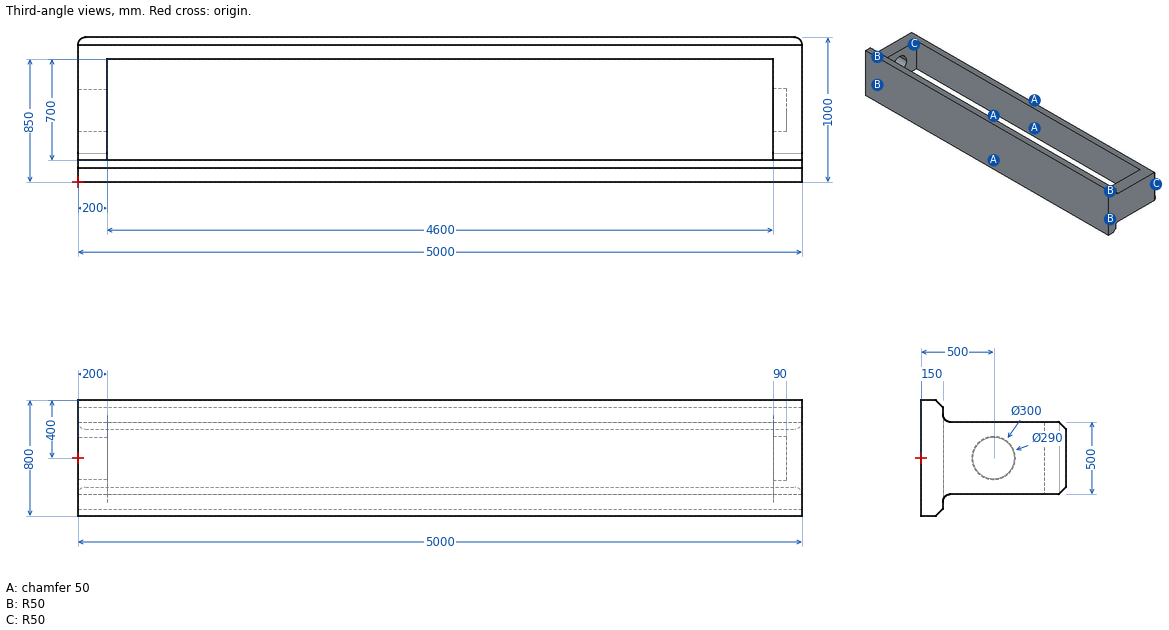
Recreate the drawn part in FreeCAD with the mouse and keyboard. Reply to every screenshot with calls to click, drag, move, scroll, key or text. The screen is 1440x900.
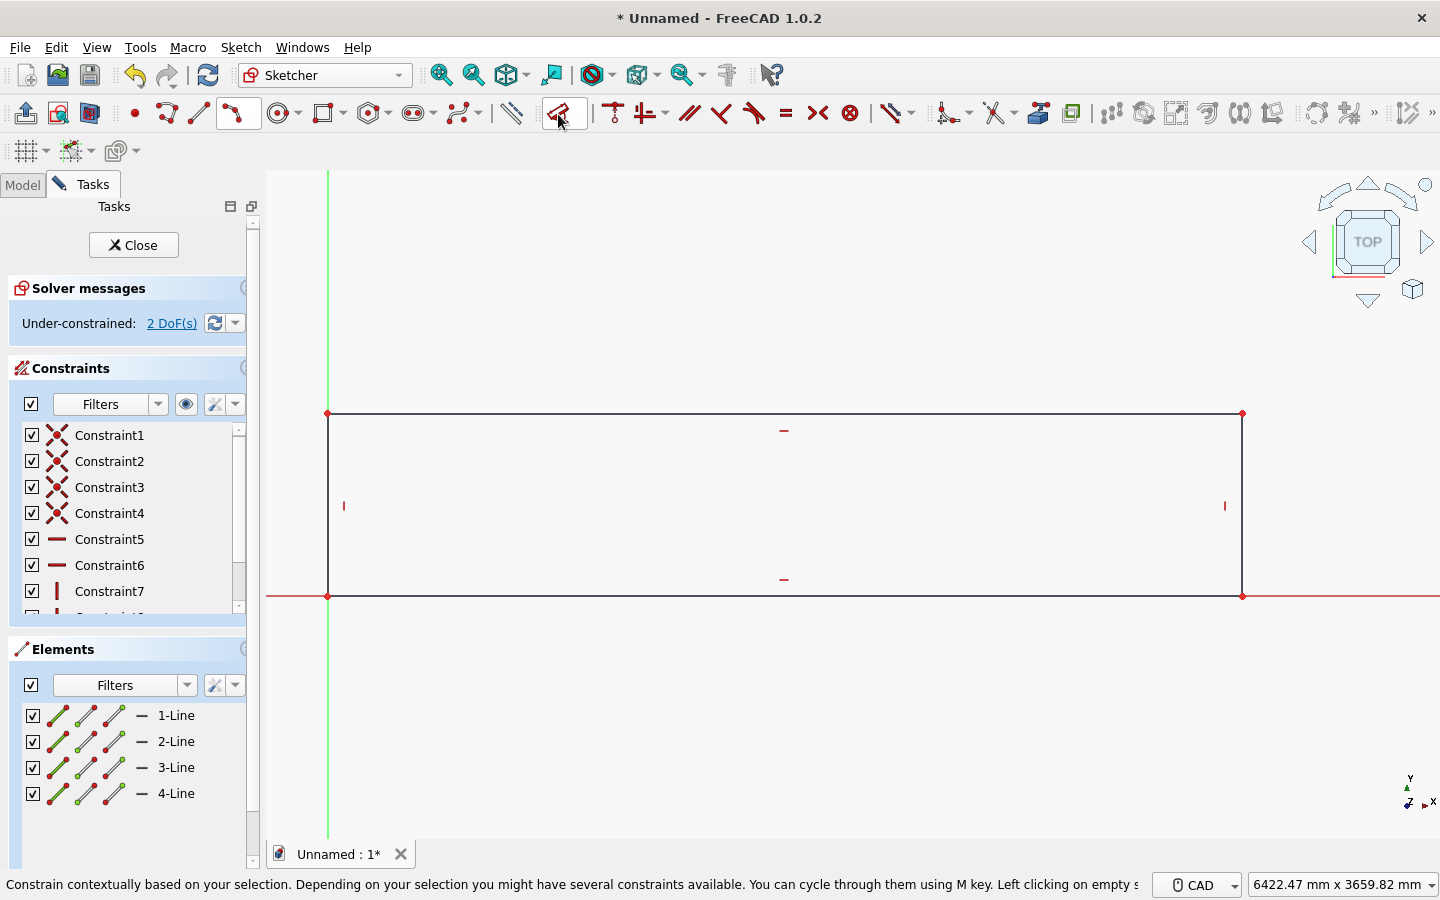
click(602, 596)
click(785, 630)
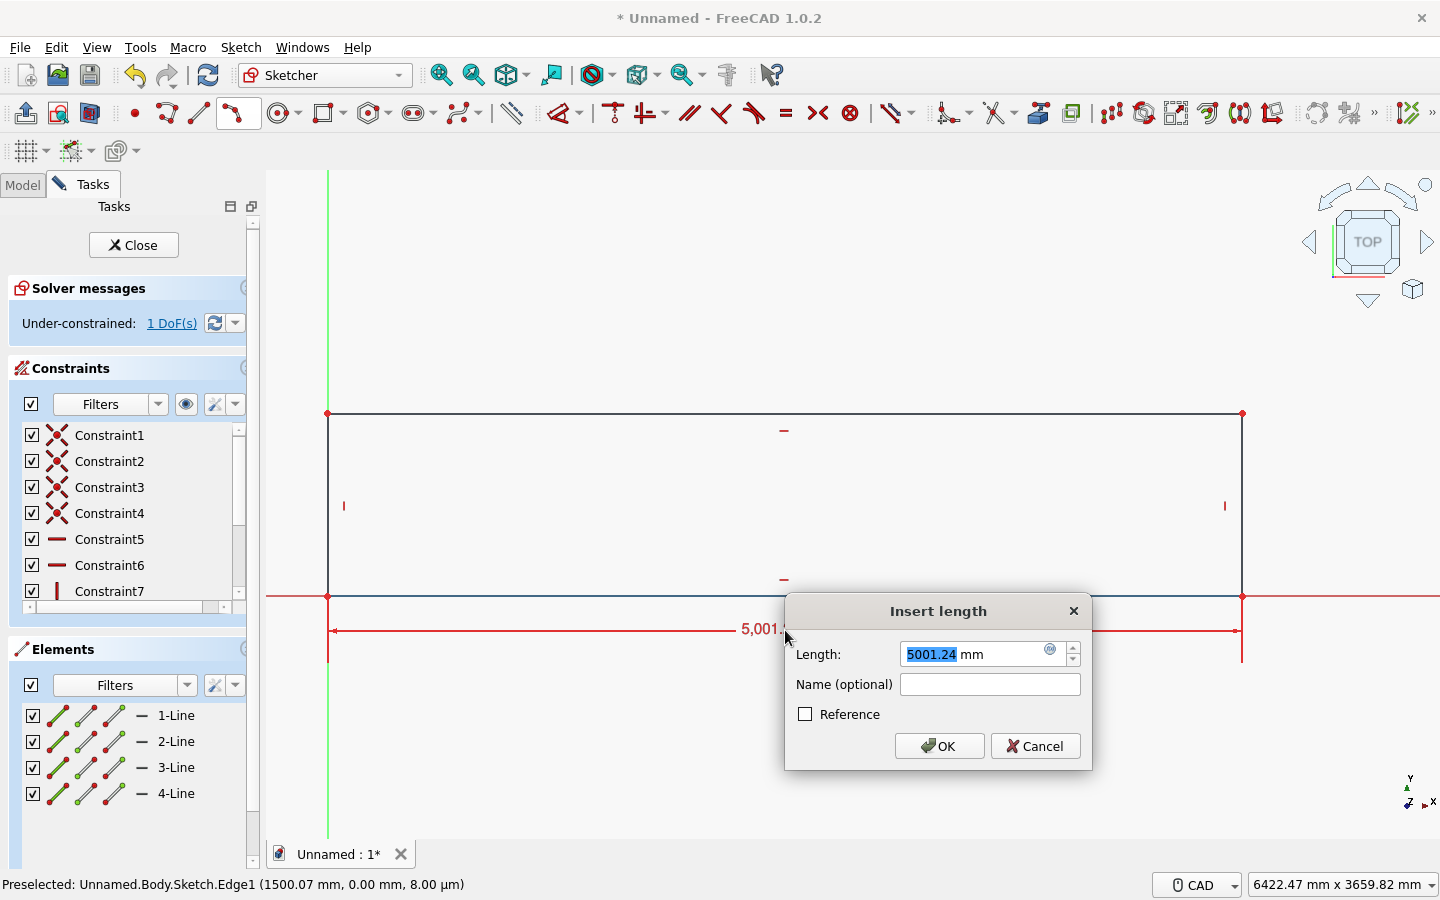
text(5000)
key(Return)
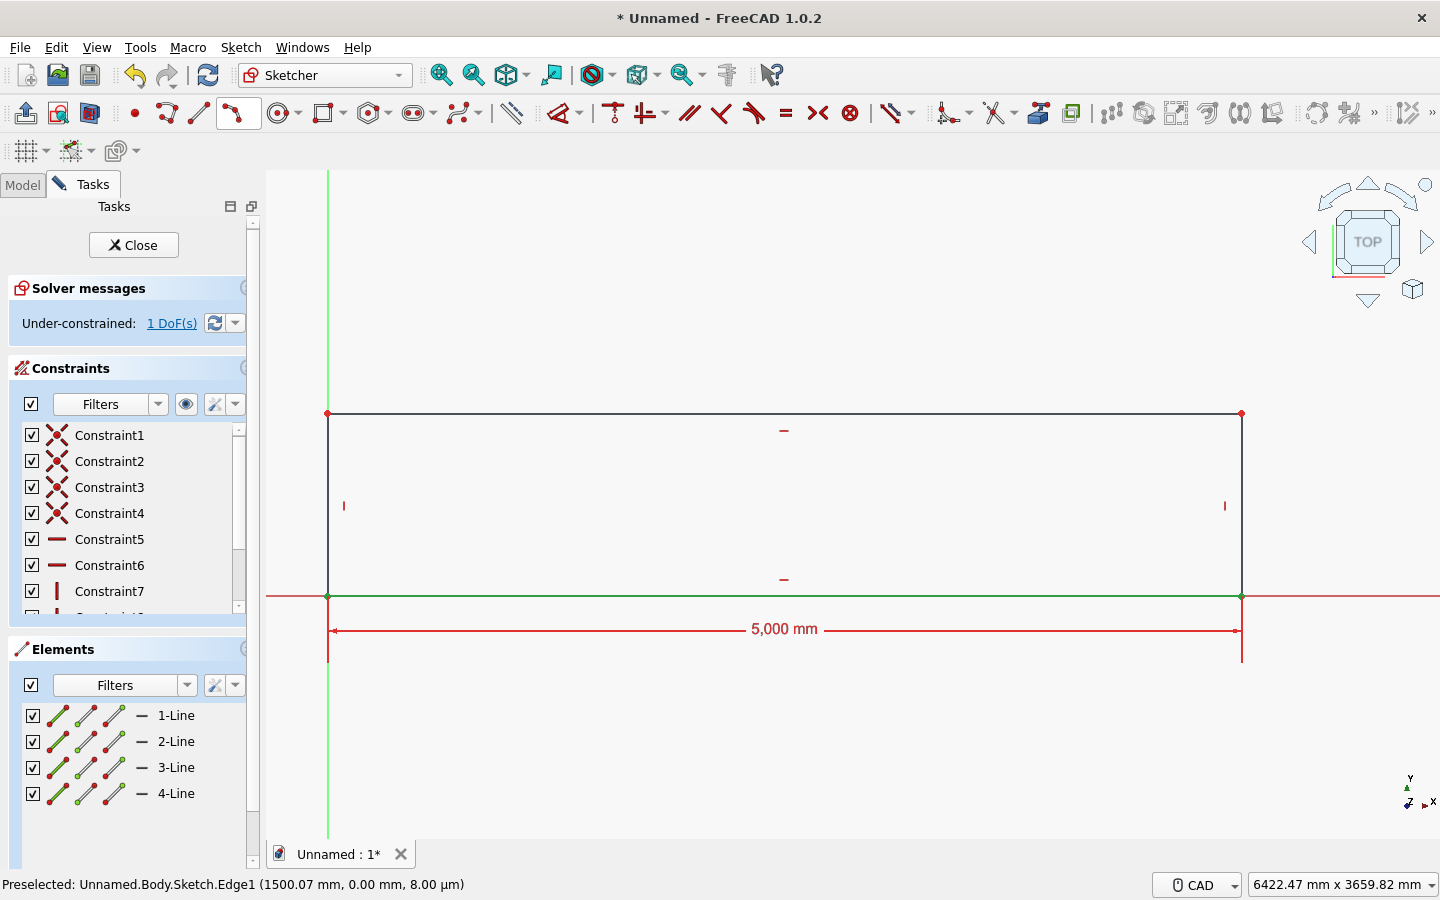
click(1242, 541)
click(1208, 505)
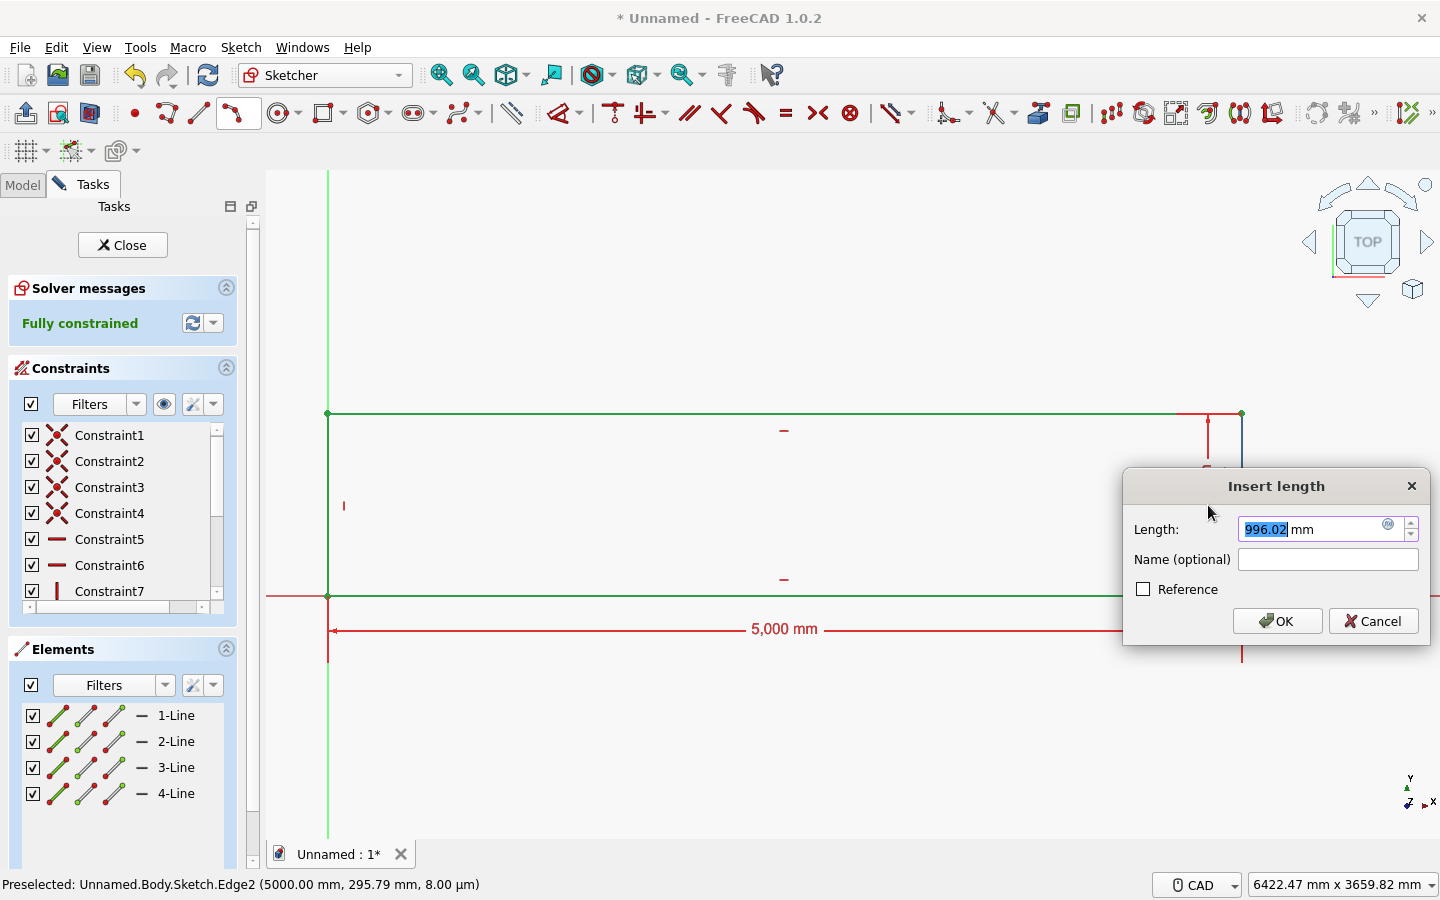
text(1000)
key(Return)
key(Escape)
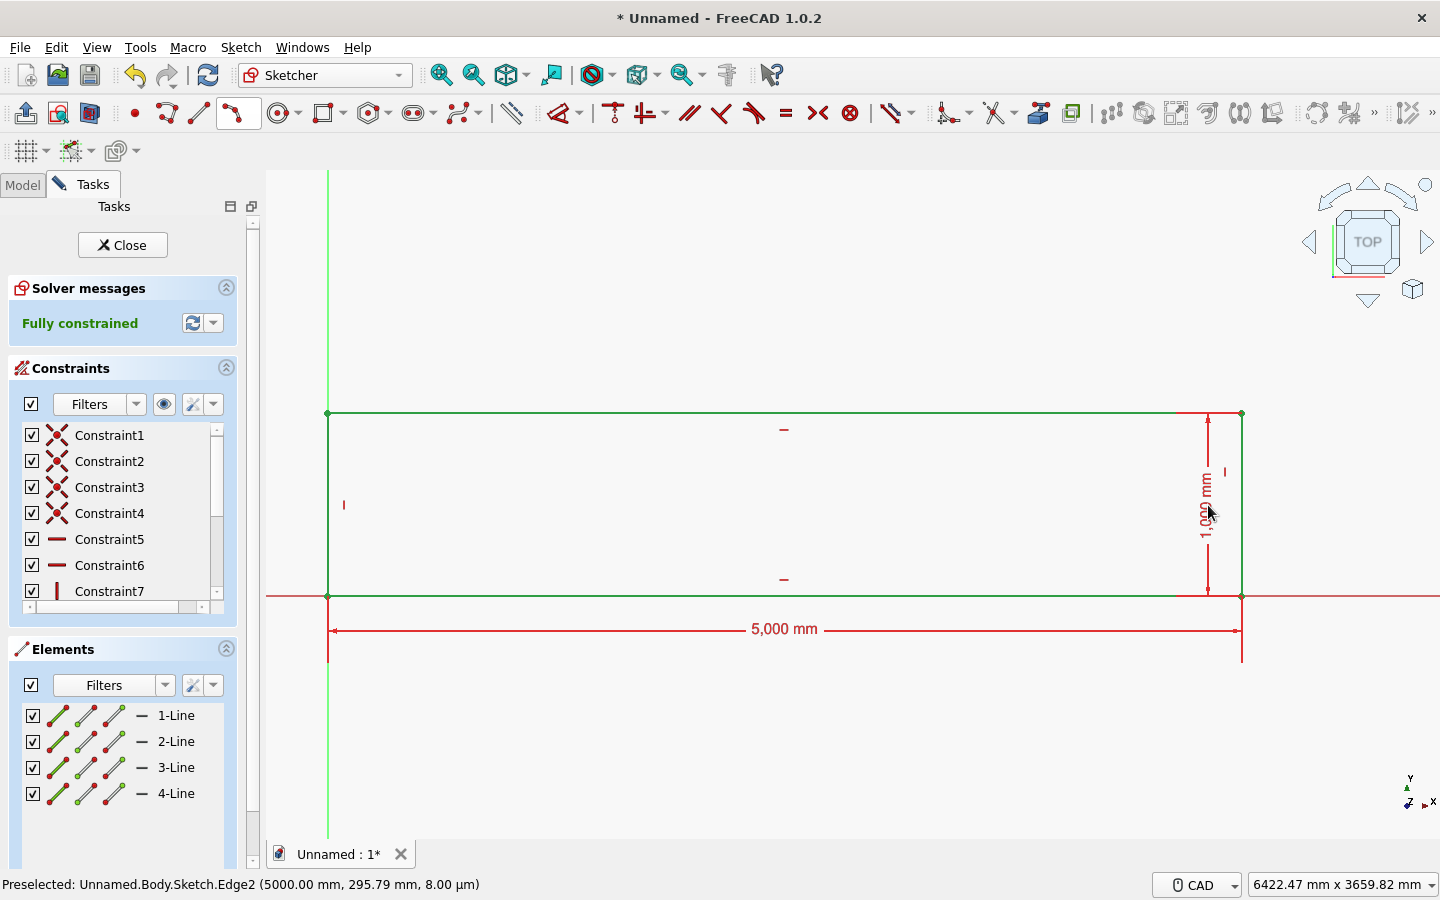
click(123, 245)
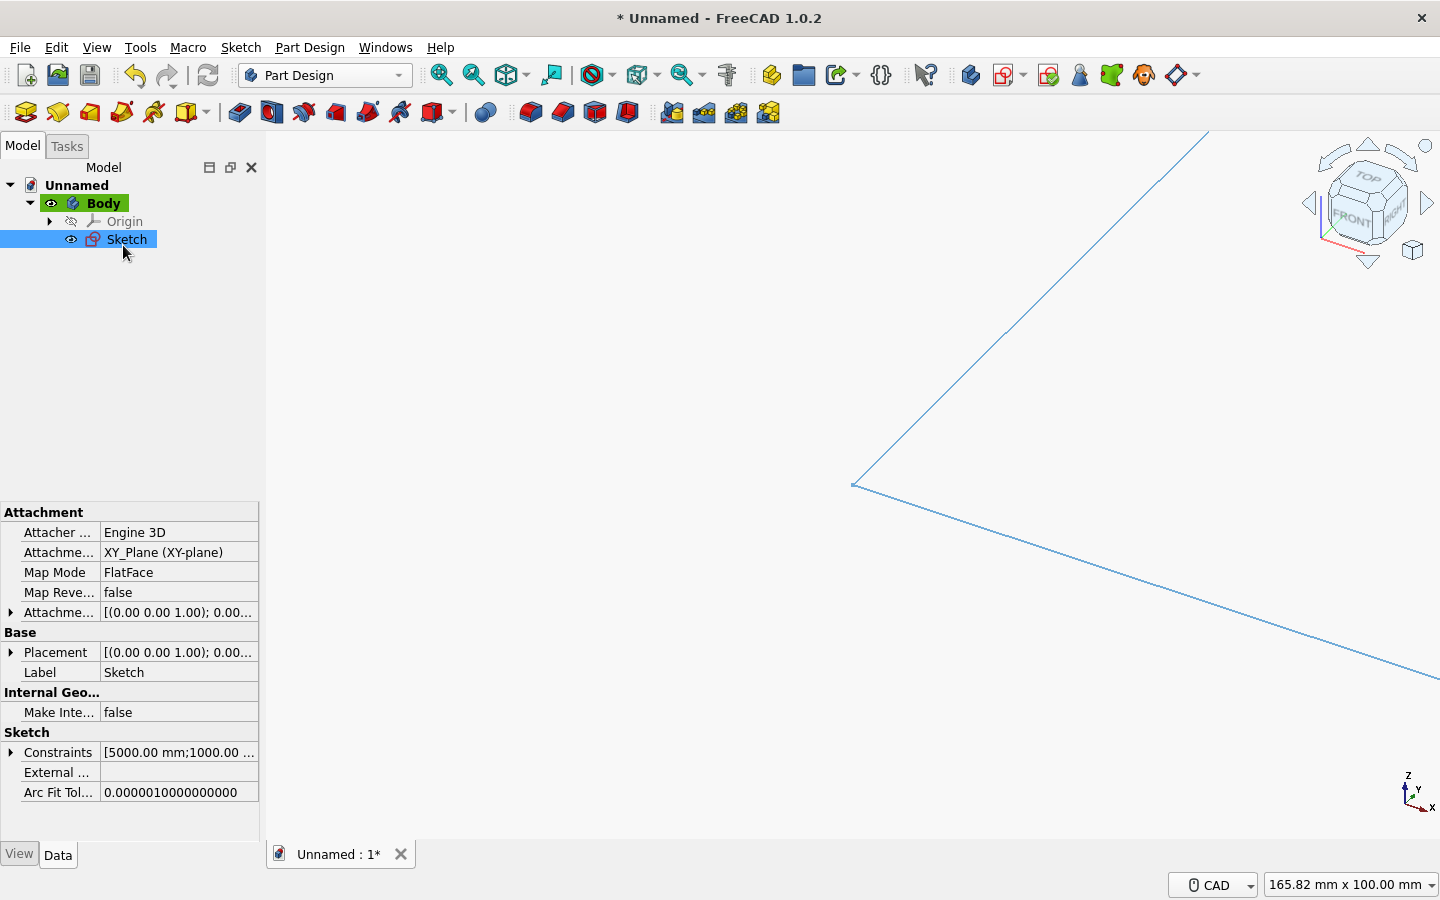
click(26, 112)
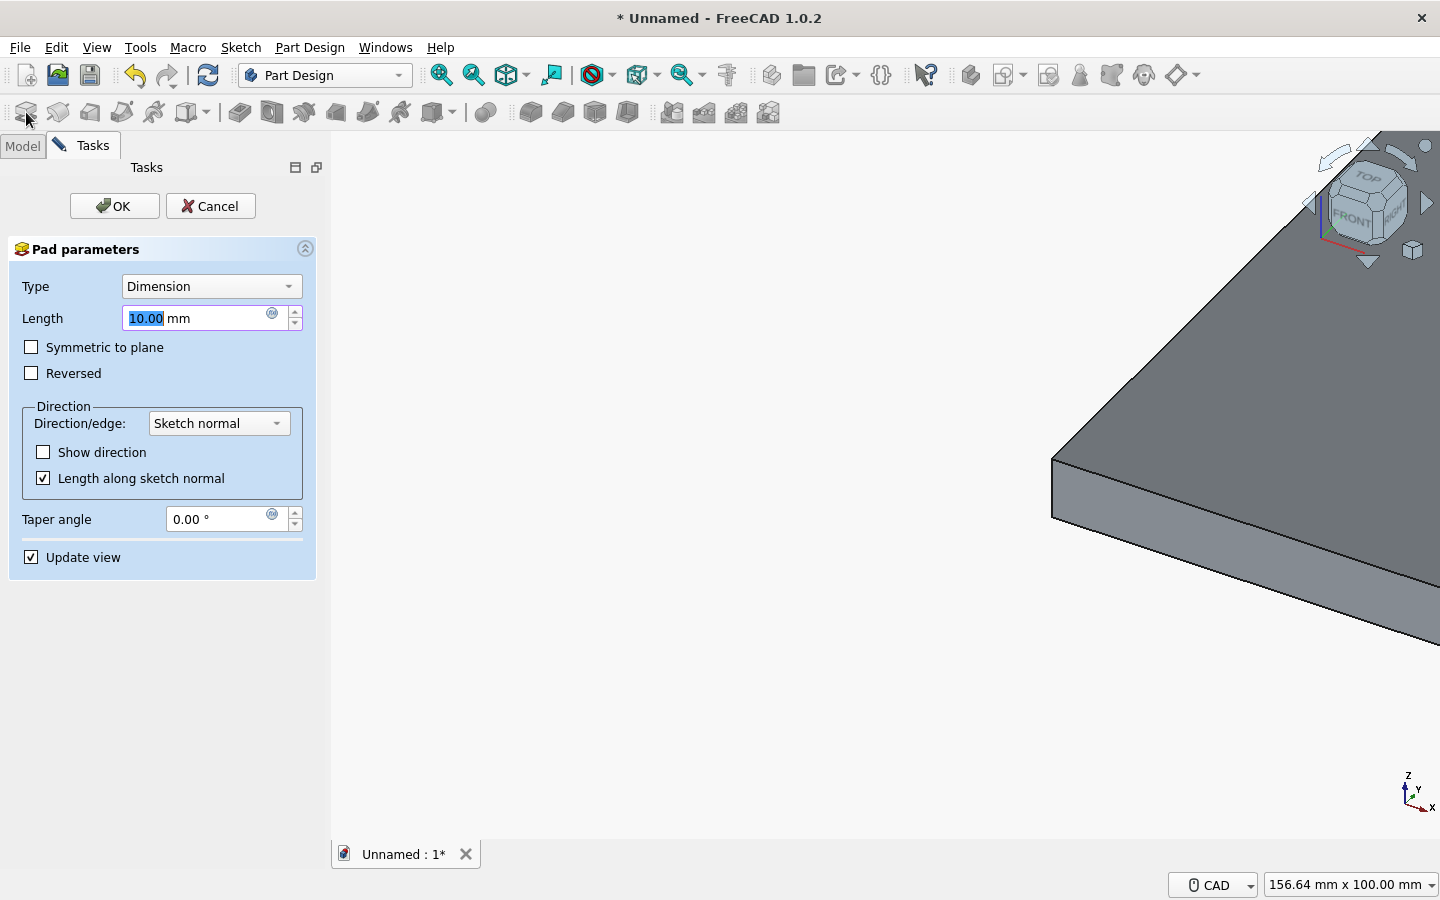
text(500)
key(Tab)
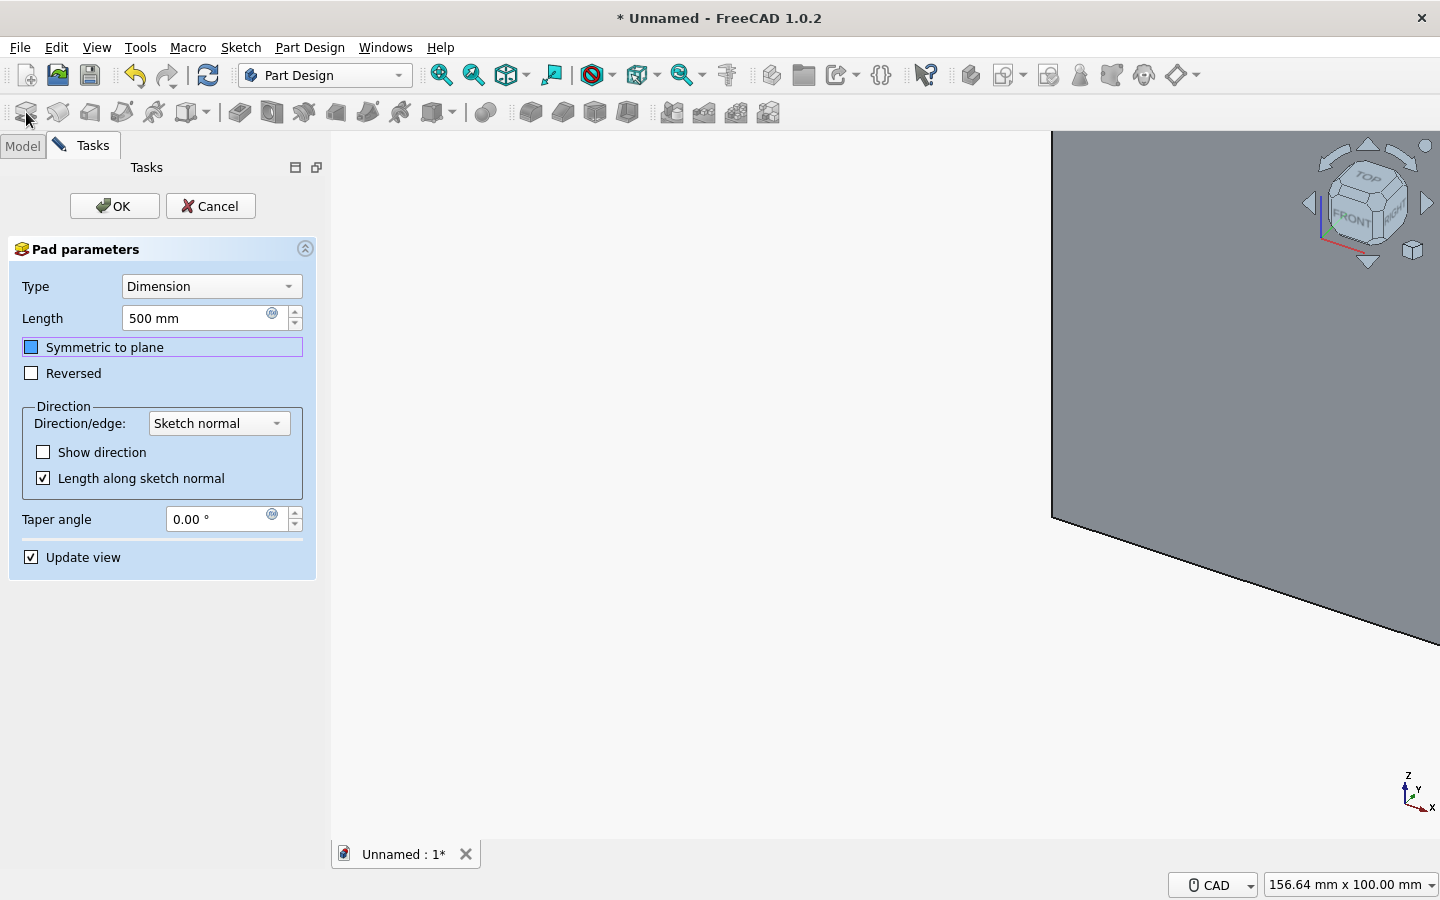
click(30, 347)